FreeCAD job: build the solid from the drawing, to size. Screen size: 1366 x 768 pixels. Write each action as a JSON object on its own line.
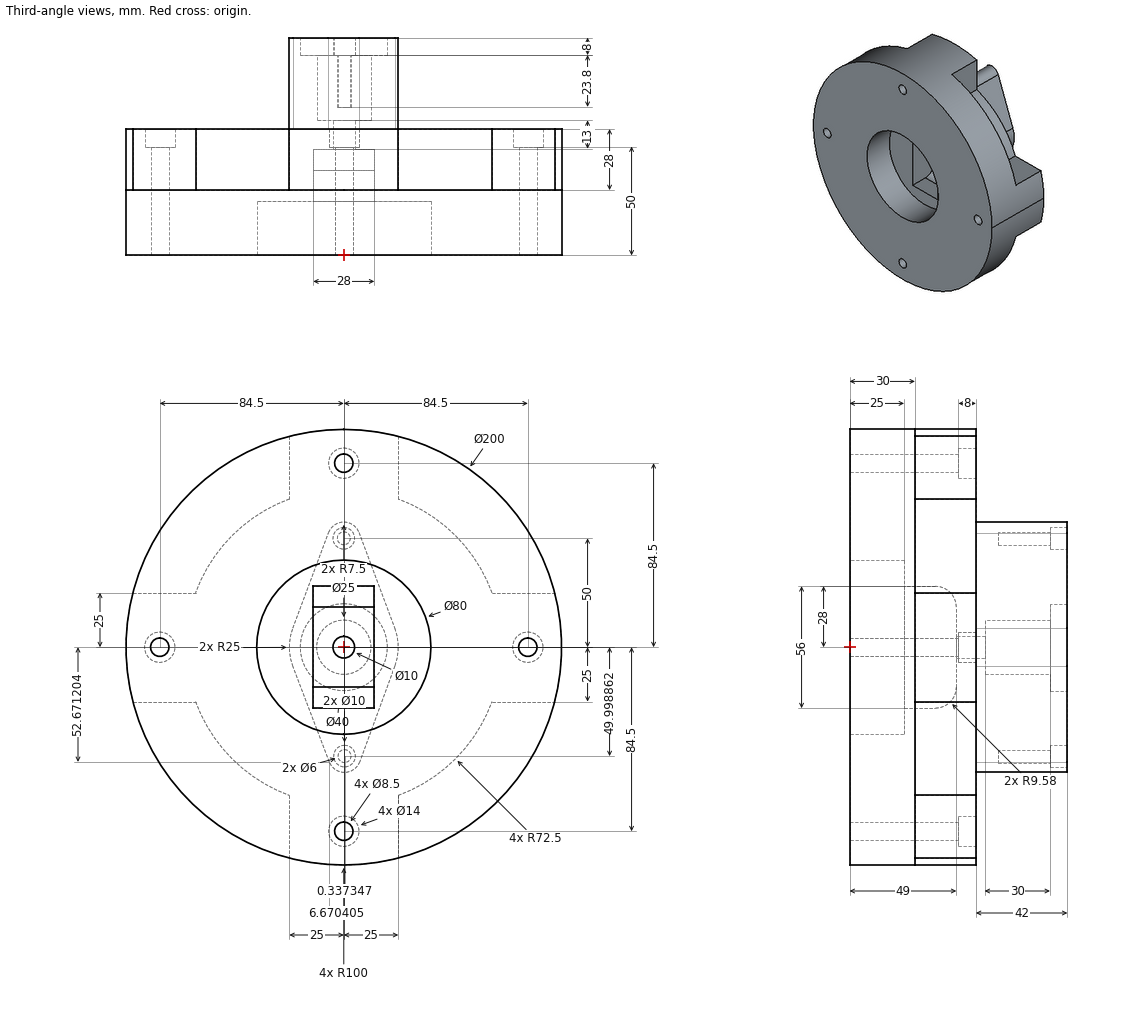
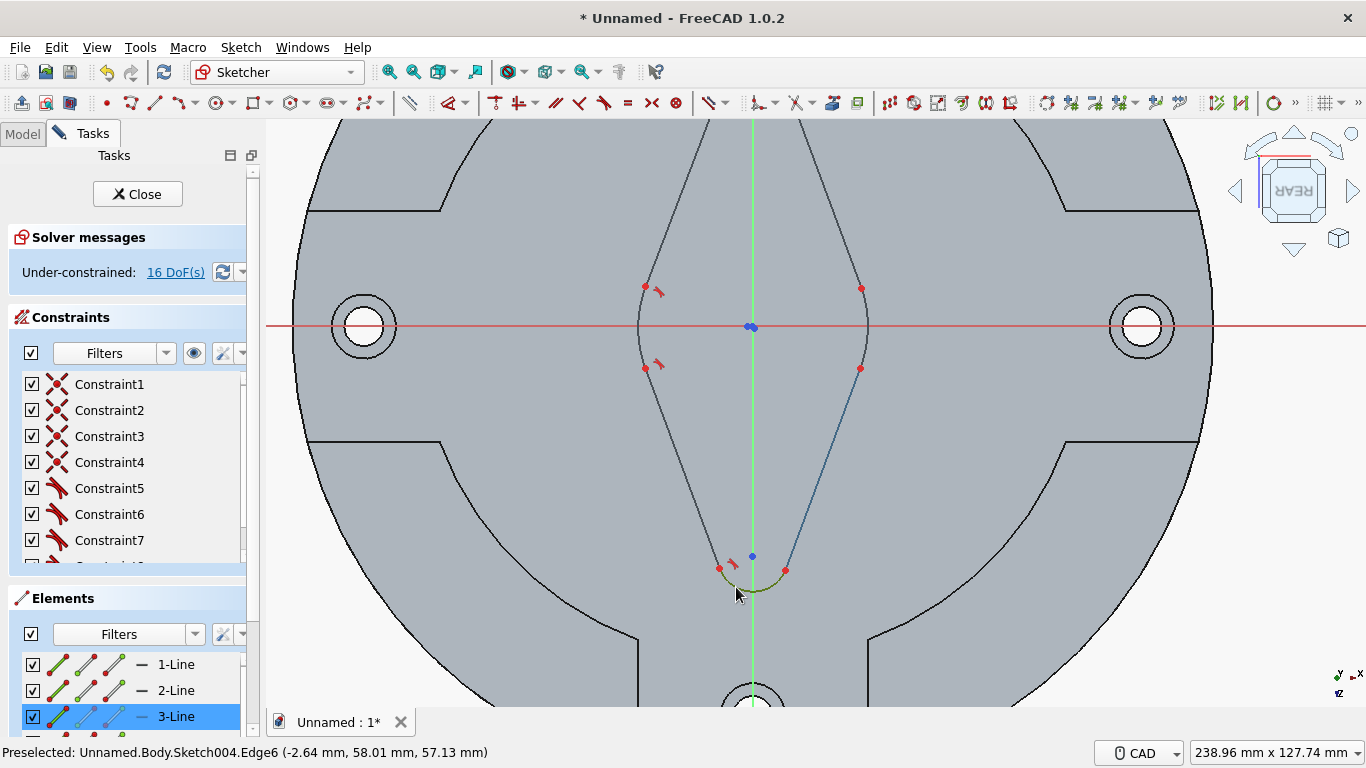
{"action": "key", "text": "t"}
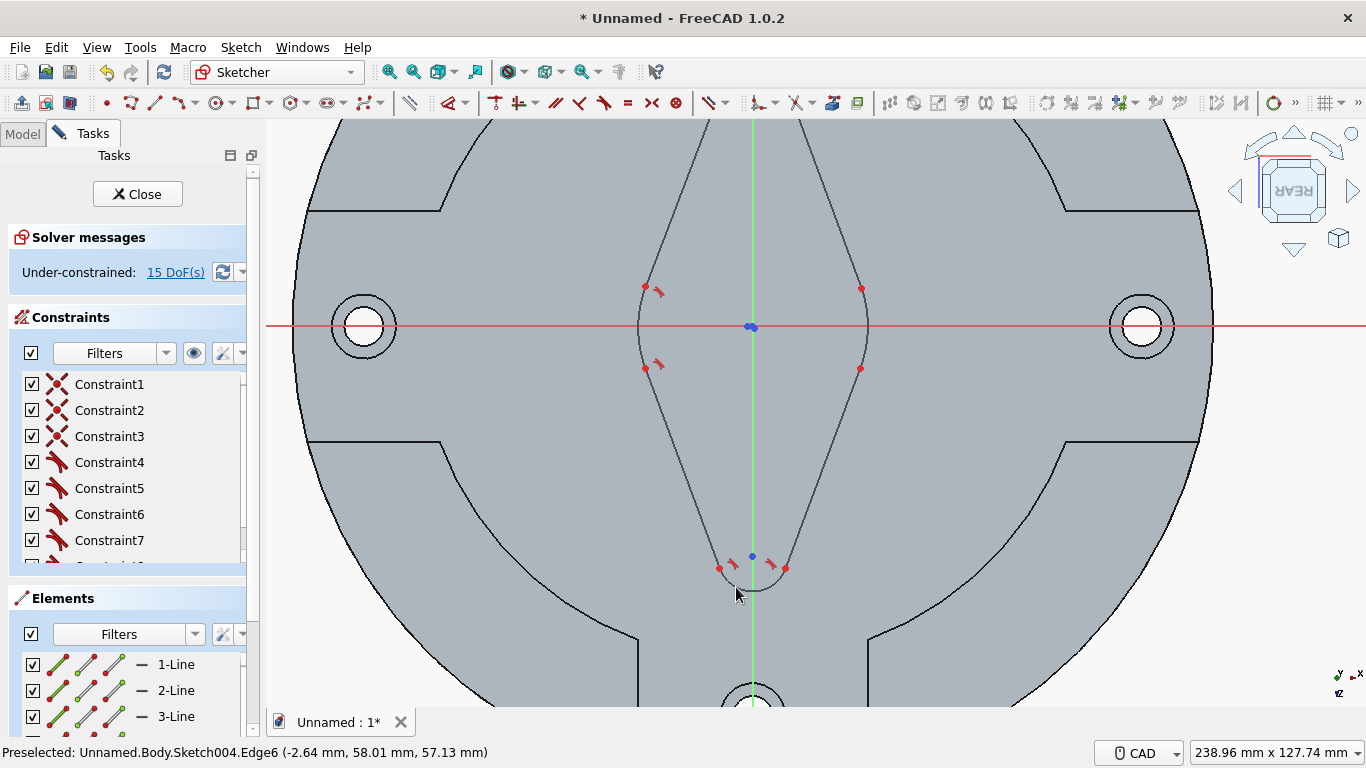
{"action": "left_click", "coordinate": [808, 509]}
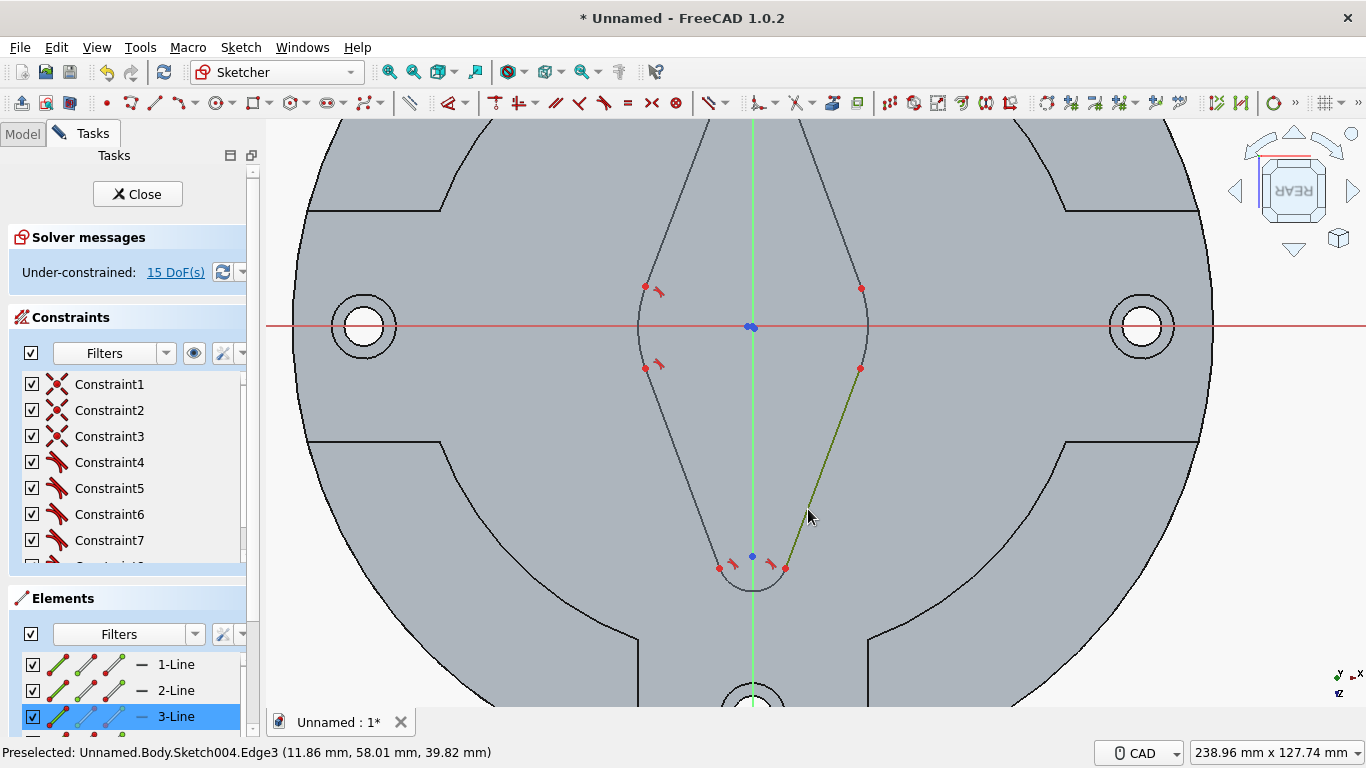
{"action": "left_click", "coordinate": [866, 345]}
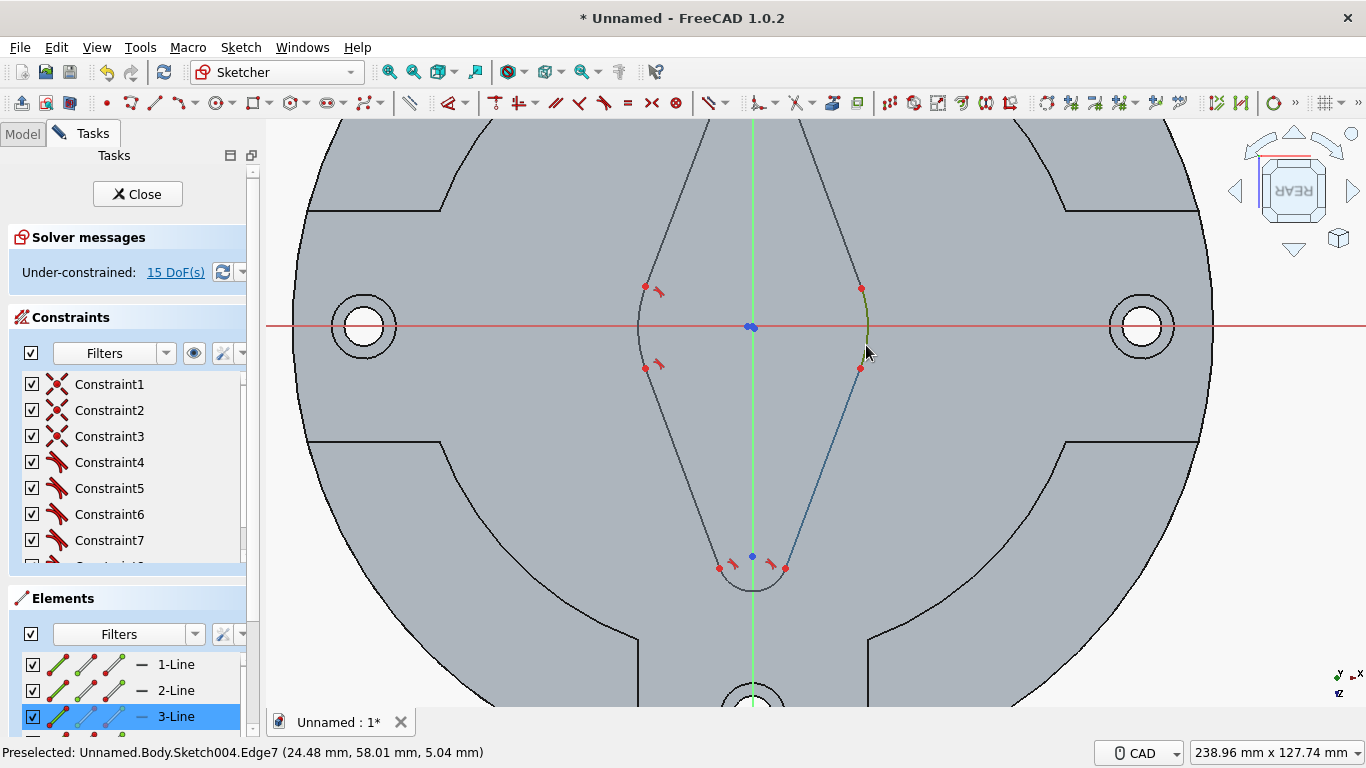
{"action": "key", "text": "t"}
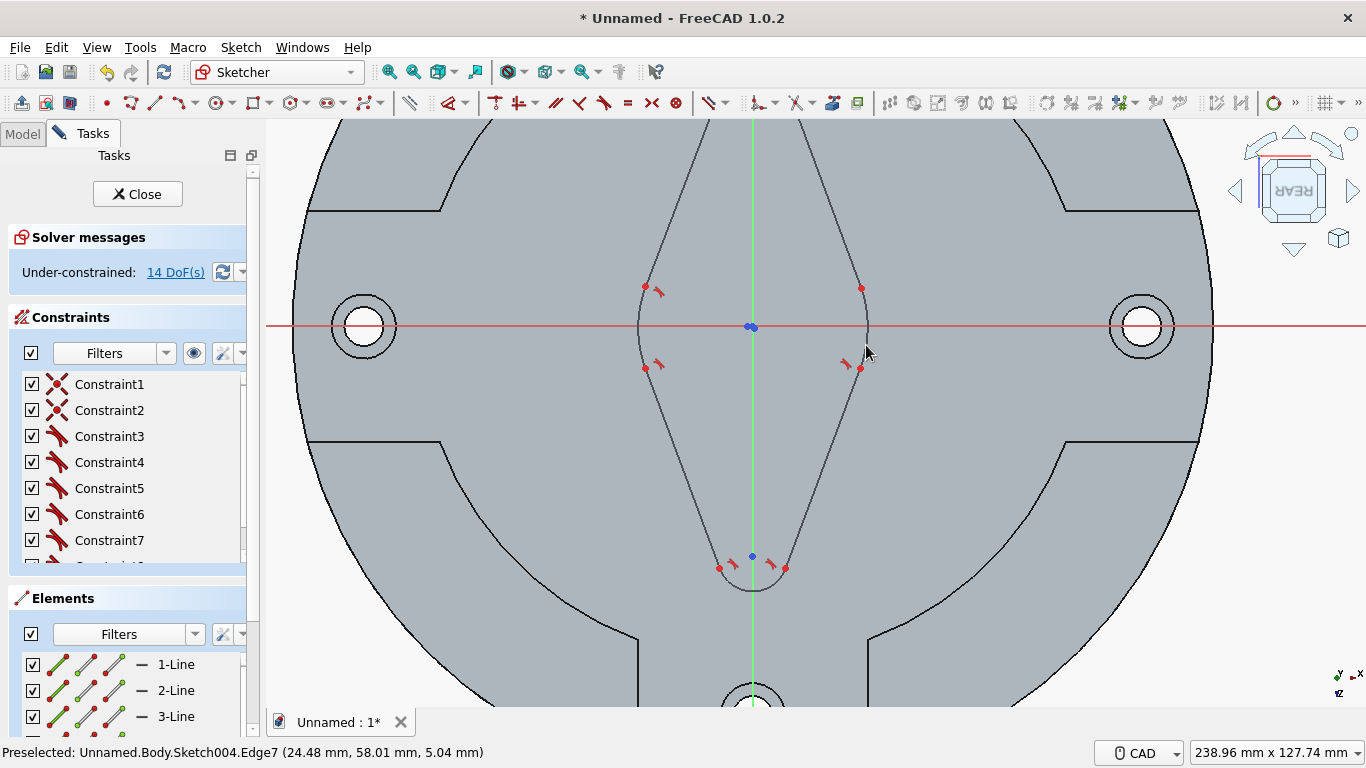
{"action": "left_click", "coordinate": [839, 228]}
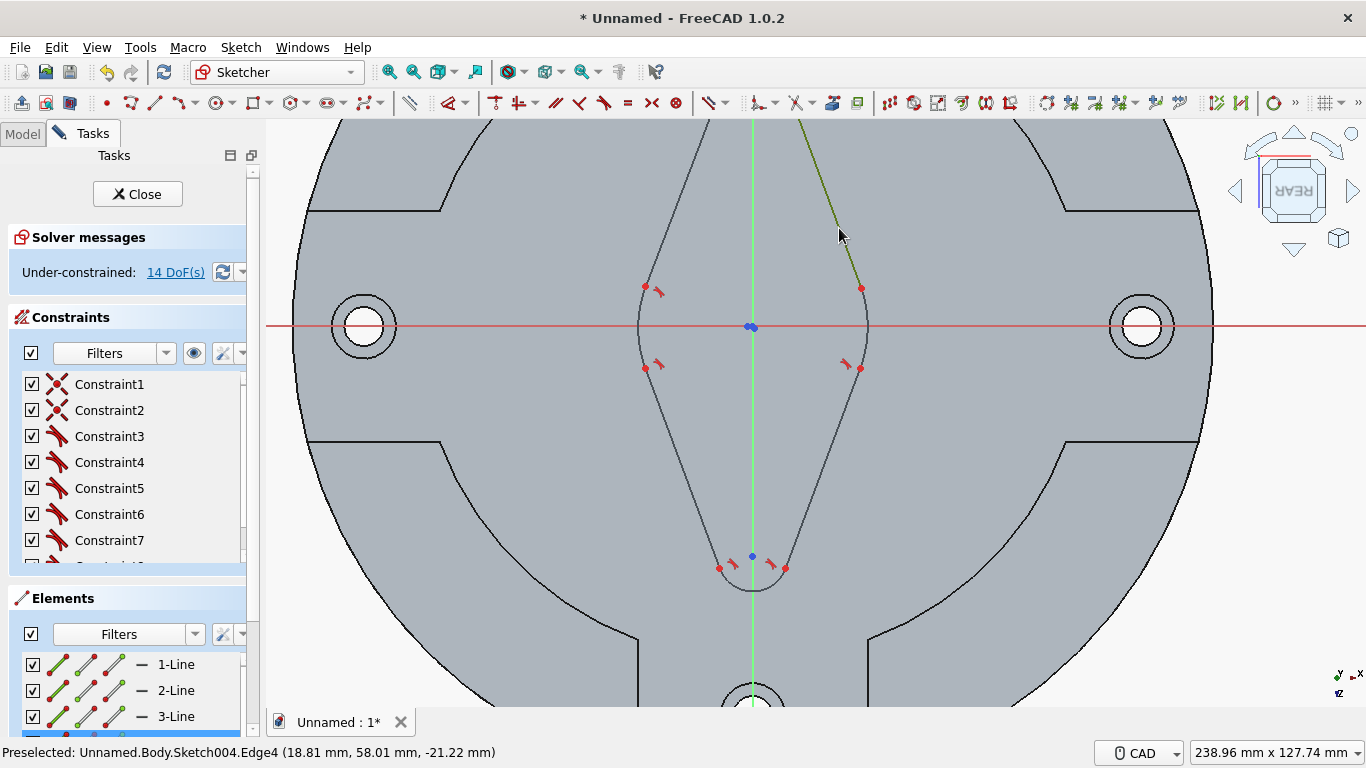
{"action": "left_click", "coordinate": [866, 345]}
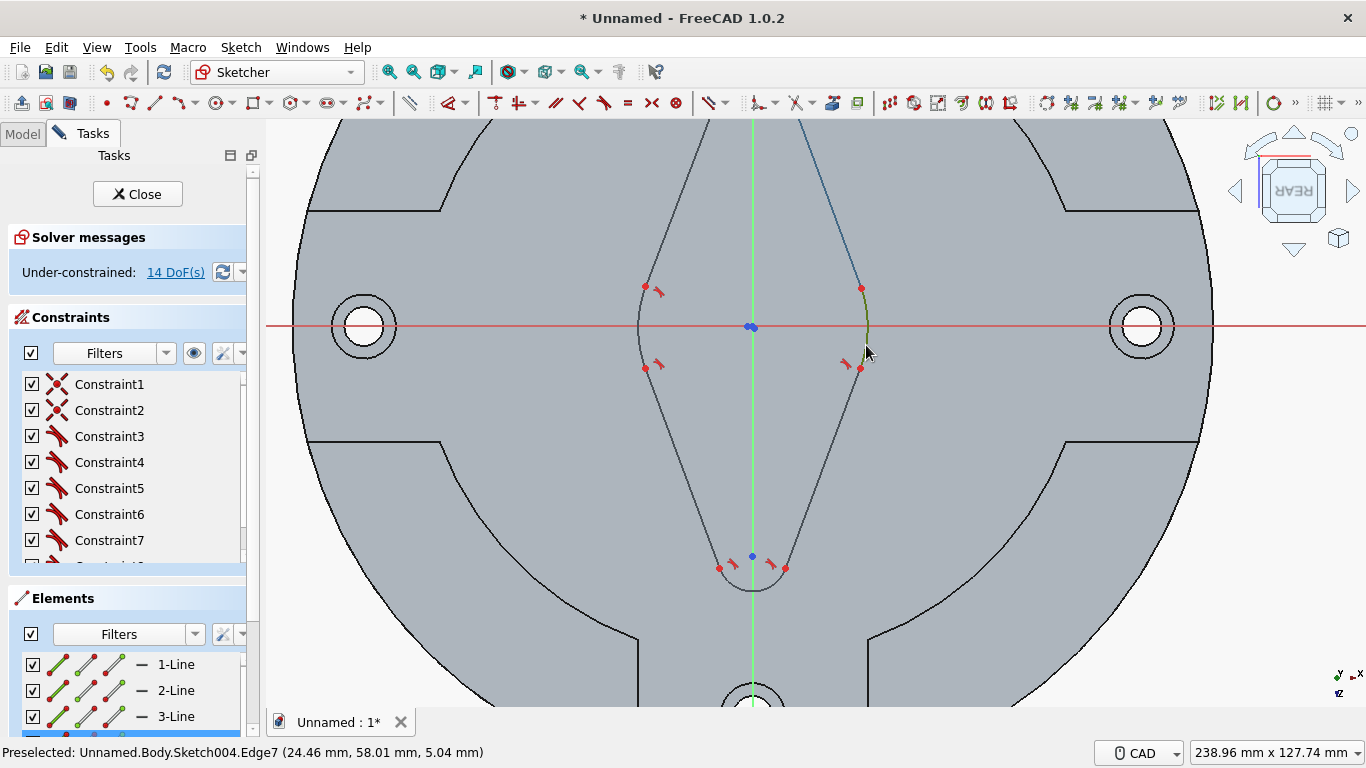
{"action": "key", "text": "t"}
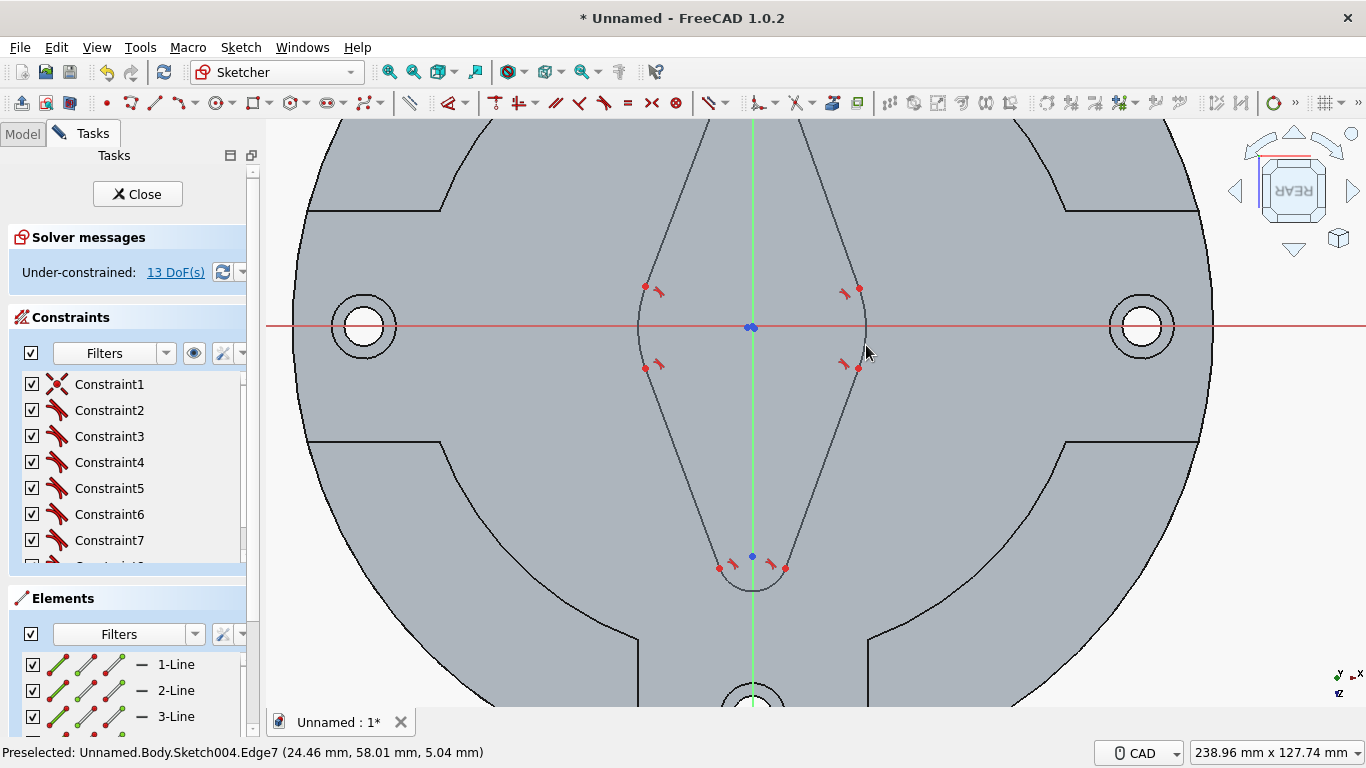
{"action": "left_click", "coordinate": [837, 228]}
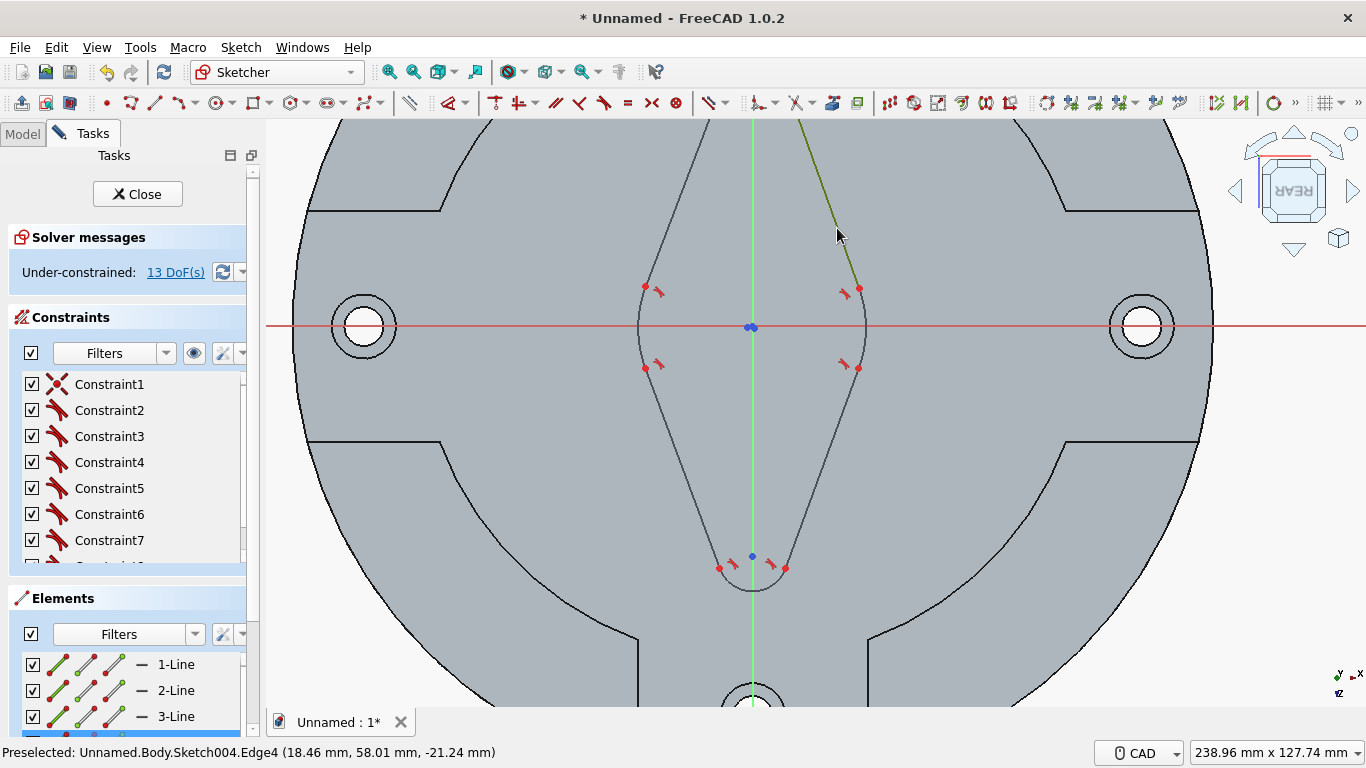
{"action": "scroll", "coordinate": [737, 589], "scroll_direction": "down", "scroll_amount": 2}